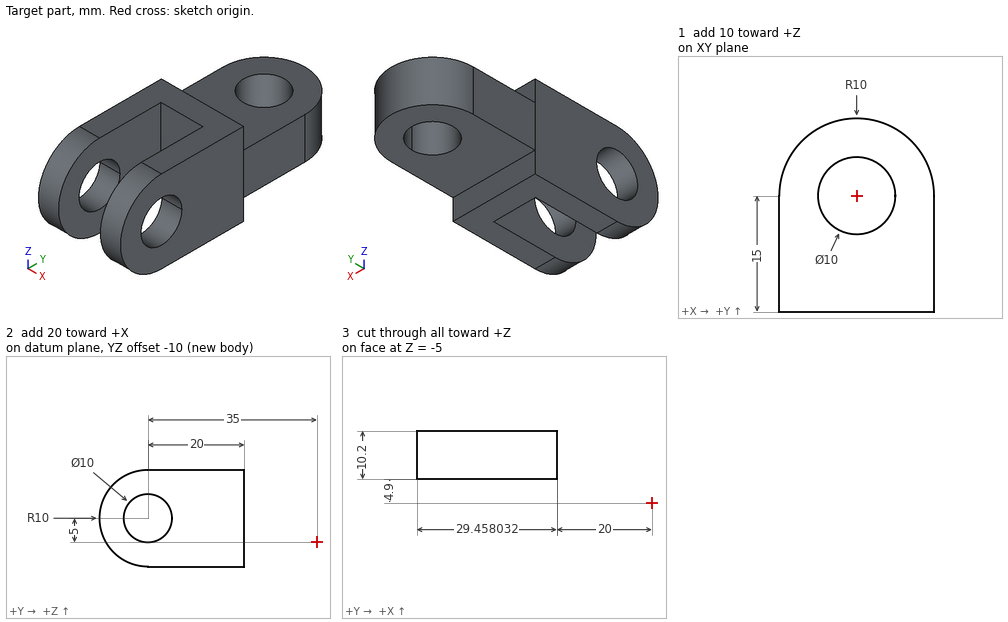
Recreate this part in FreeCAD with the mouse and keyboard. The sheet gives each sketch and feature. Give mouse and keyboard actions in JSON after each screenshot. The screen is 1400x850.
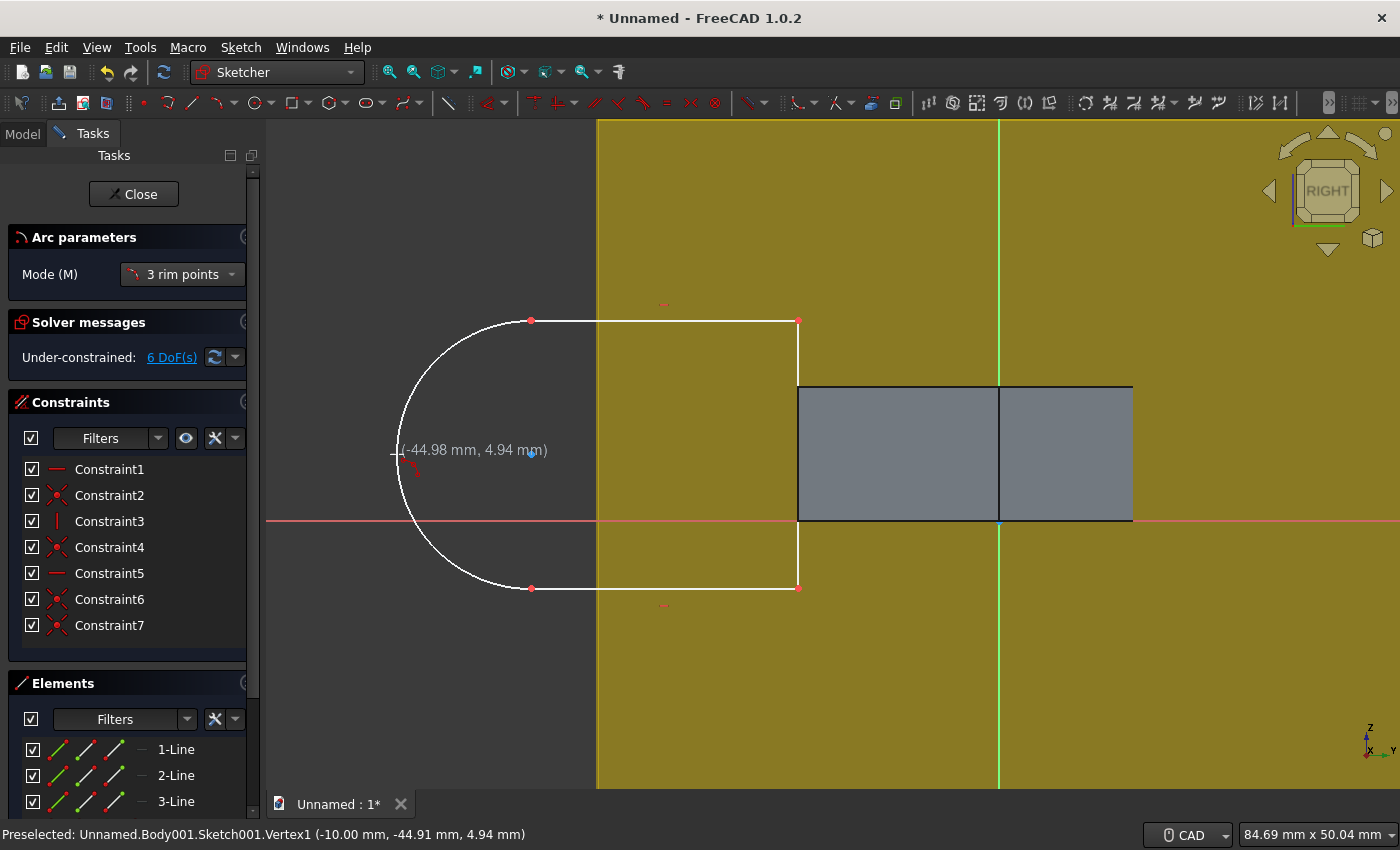
{"action": "left_click", "coordinate": [256, 104]}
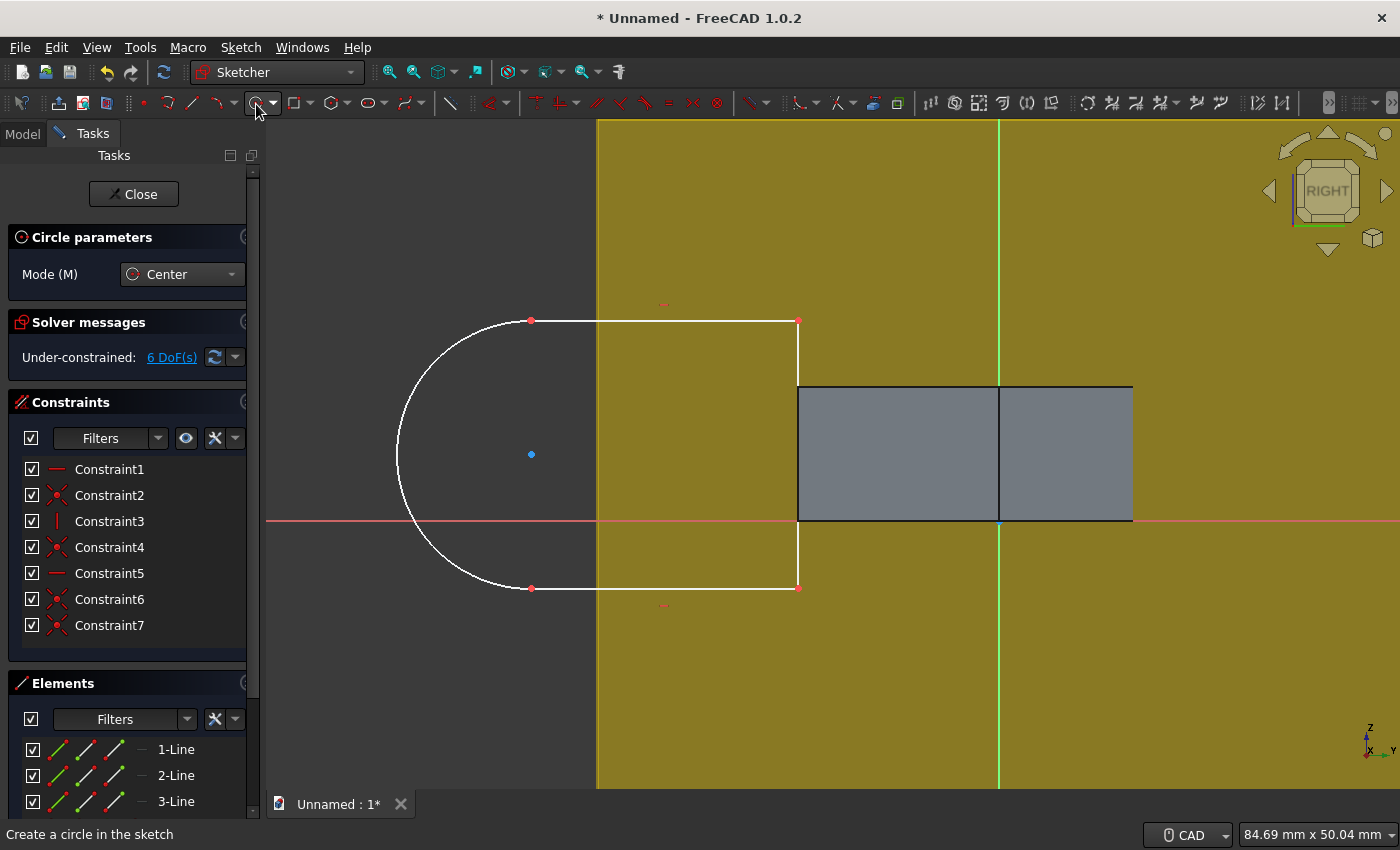
{"action": "left_click", "coordinate": [531, 454]}
{"action": "left_click", "coordinate": [578, 407]}
{"action": "key", "text": "Escape"}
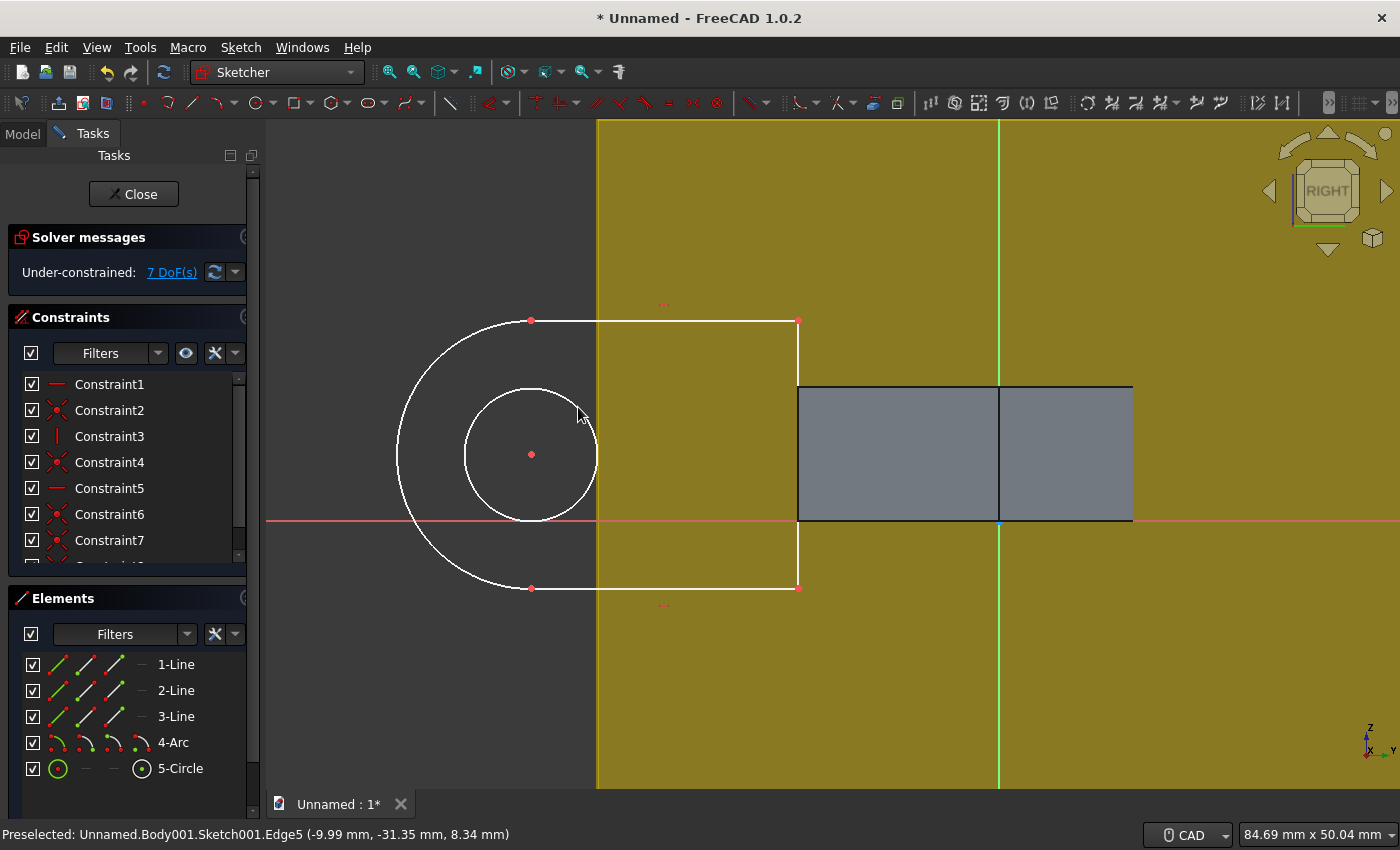
{"action": "left_click", "coordinate": [611, 321]}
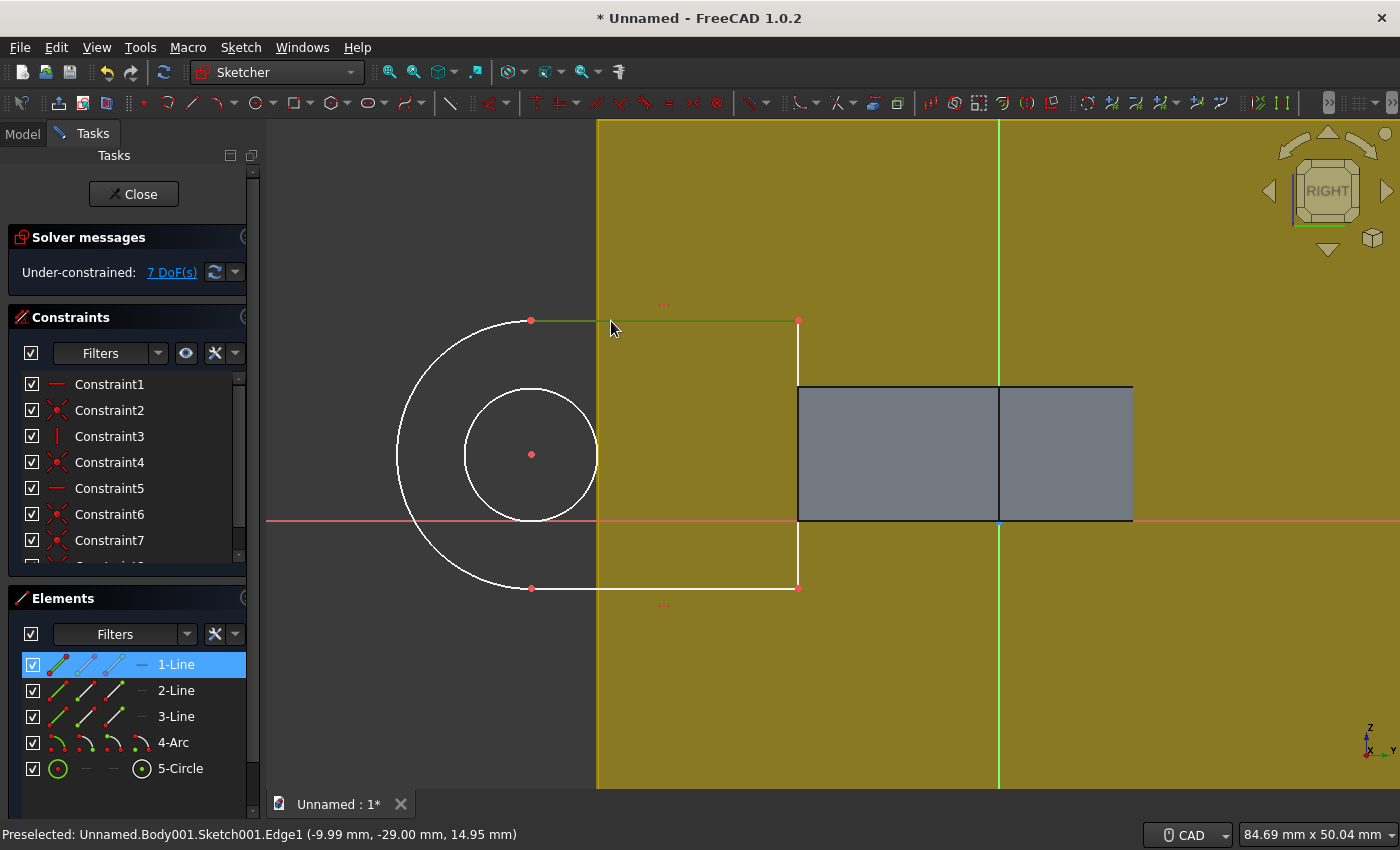
{"action": "left_click", "coordinate": [423, 376]}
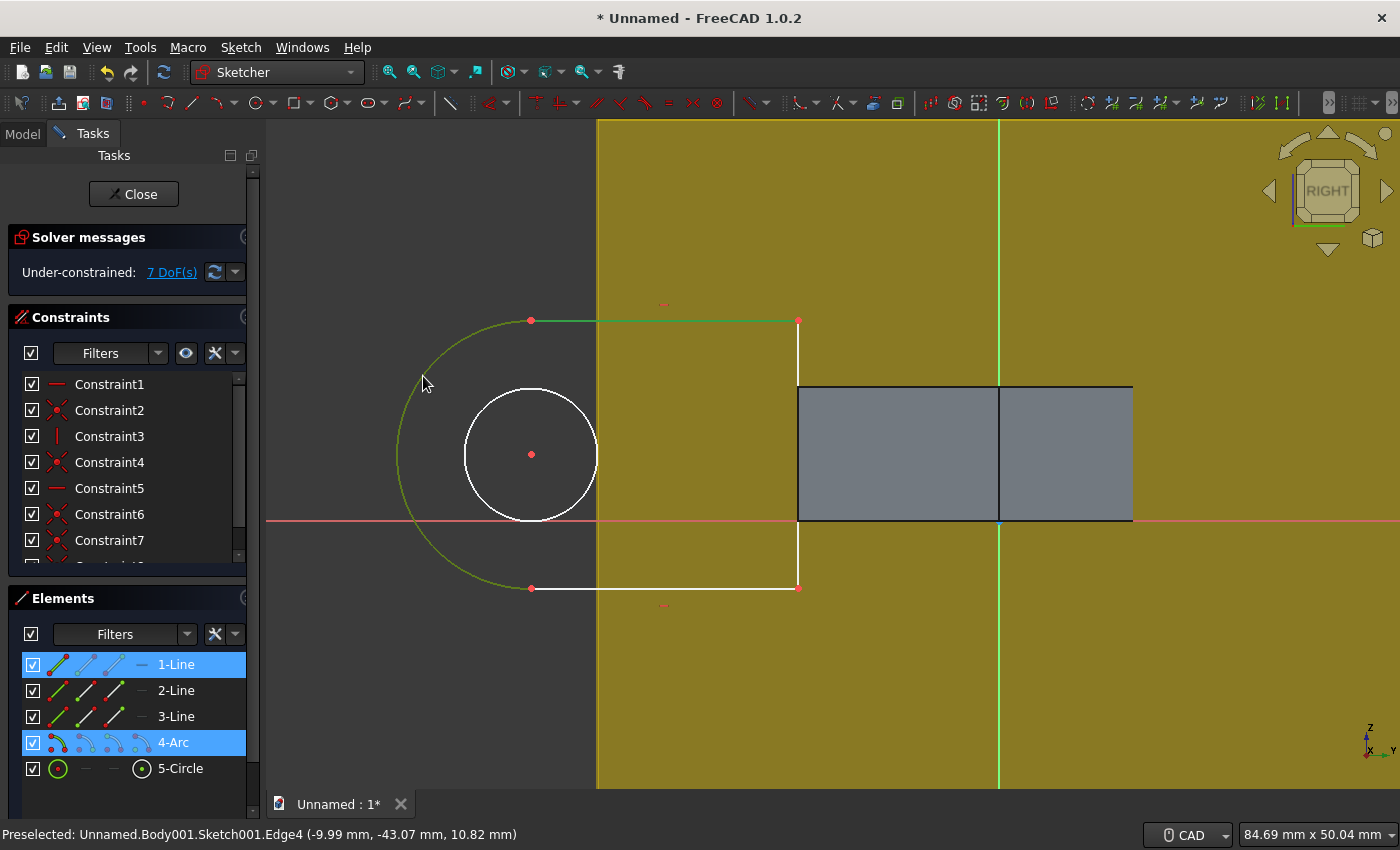
{"action": "left_click", "coordinate": [646, 104]}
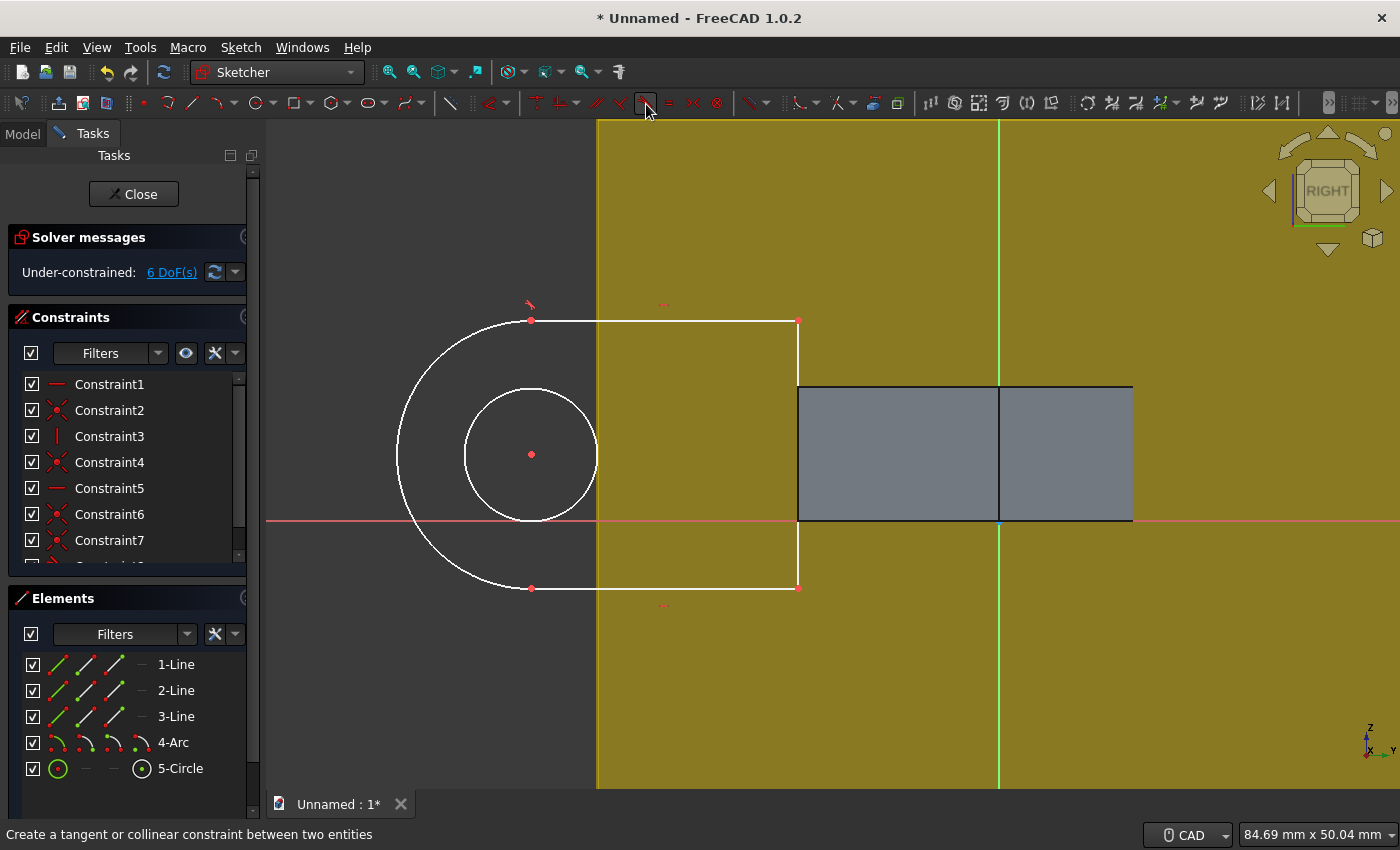
{"action": "left_click", "coordinate": [718, 589]}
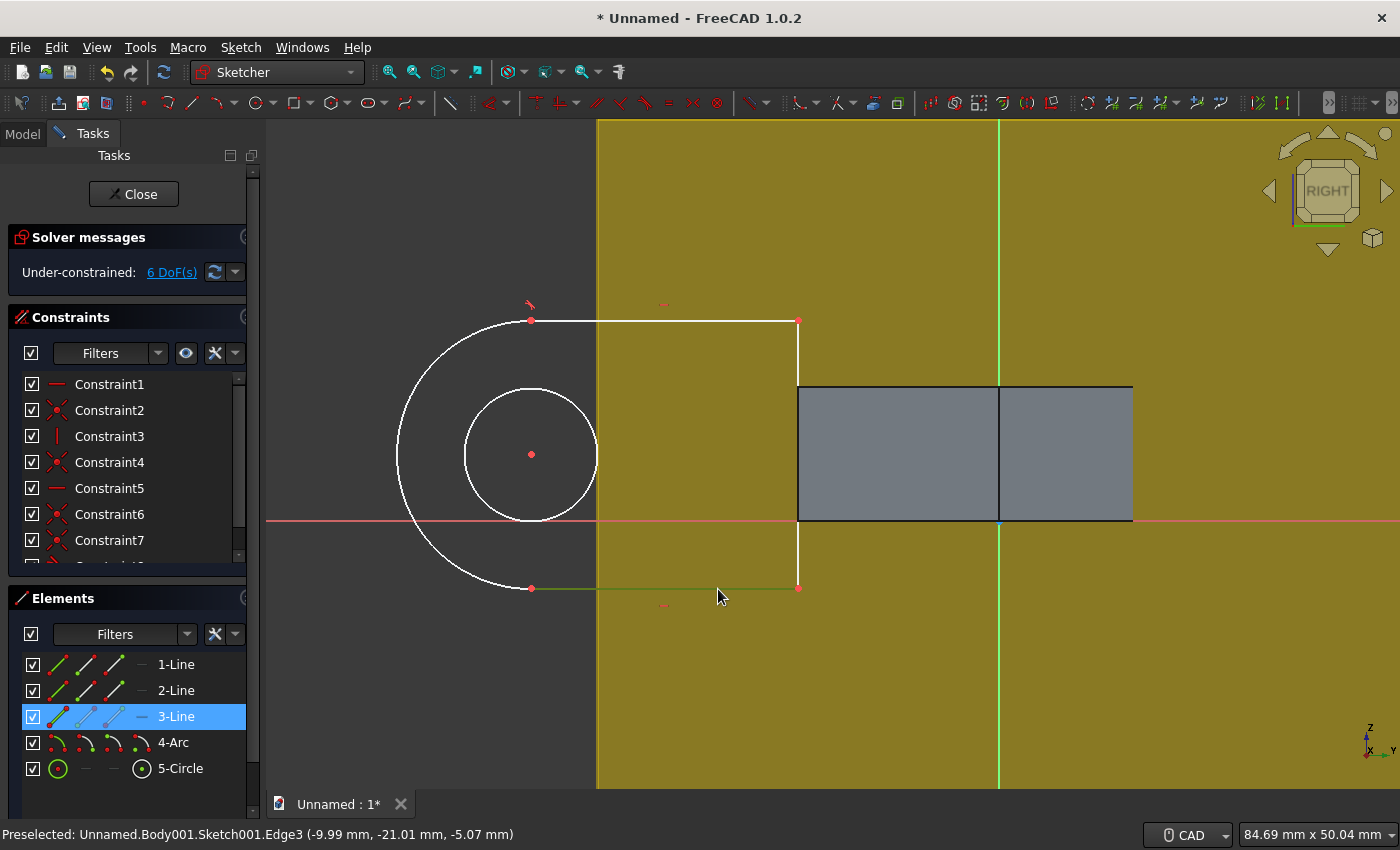
{"action": "left_click", "coordinate": [423, 376]}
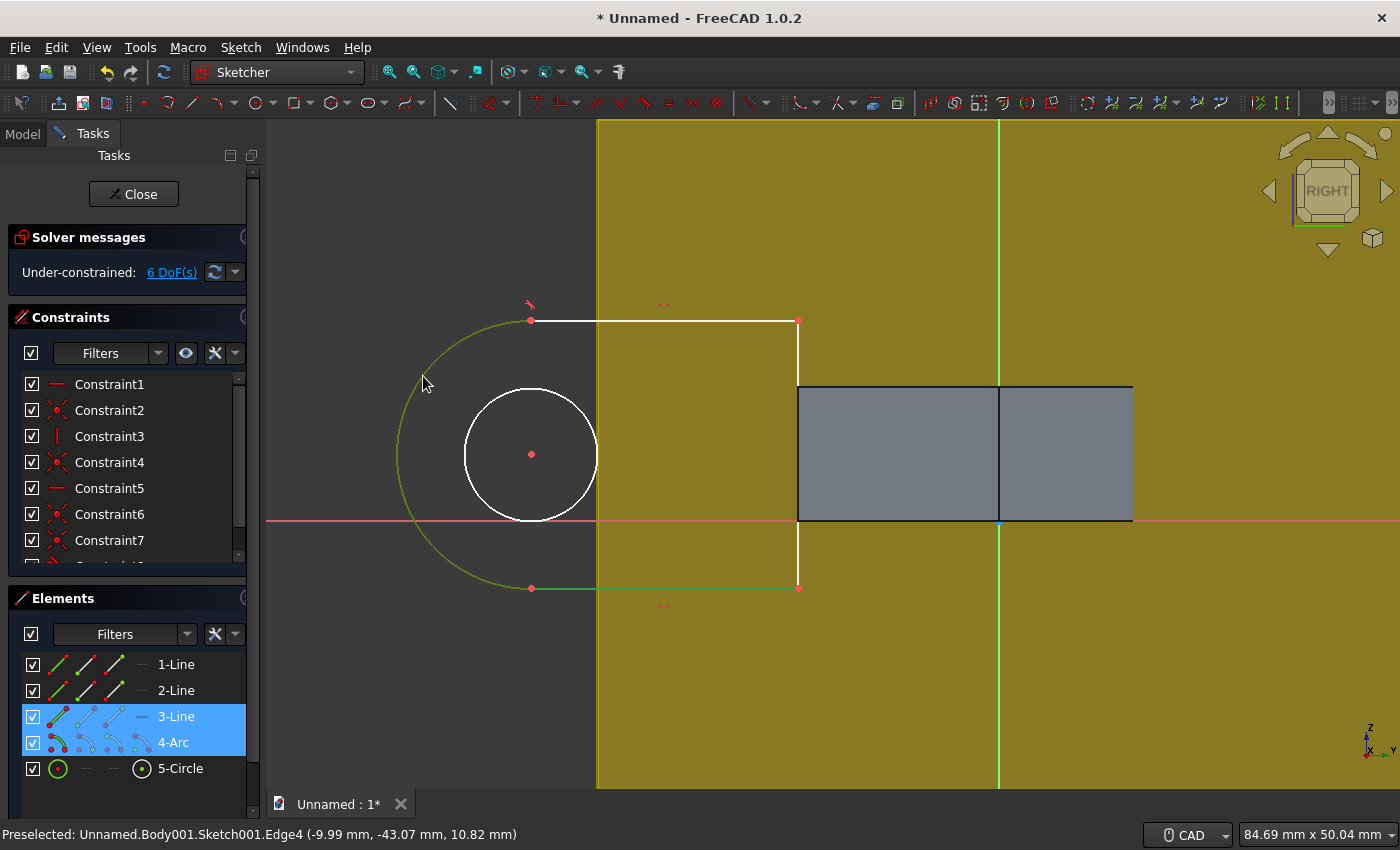
{"action": "left_click", "coordinate": [646, 104]}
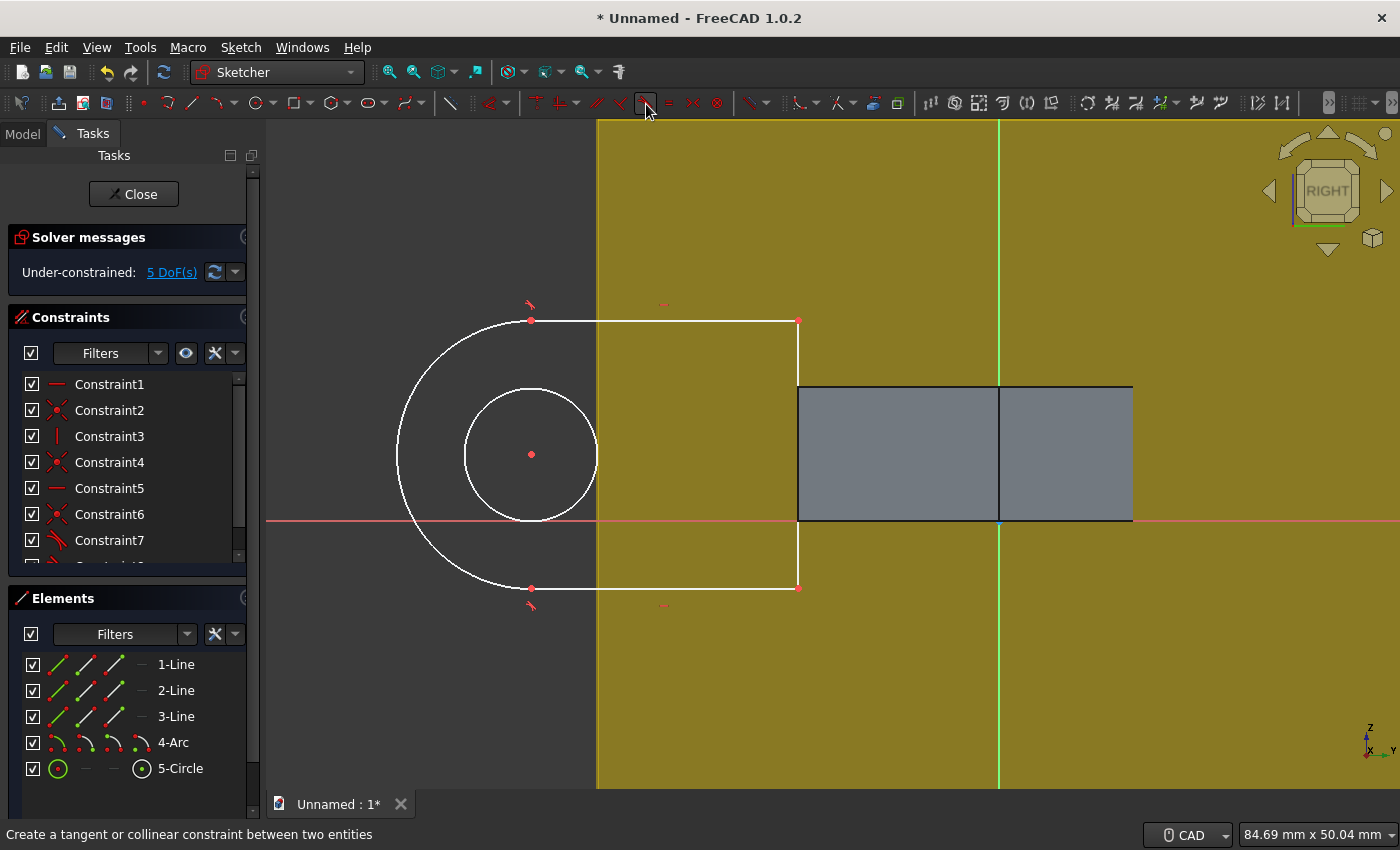
{"action": "left_click", "coordinate": [490, 104]}